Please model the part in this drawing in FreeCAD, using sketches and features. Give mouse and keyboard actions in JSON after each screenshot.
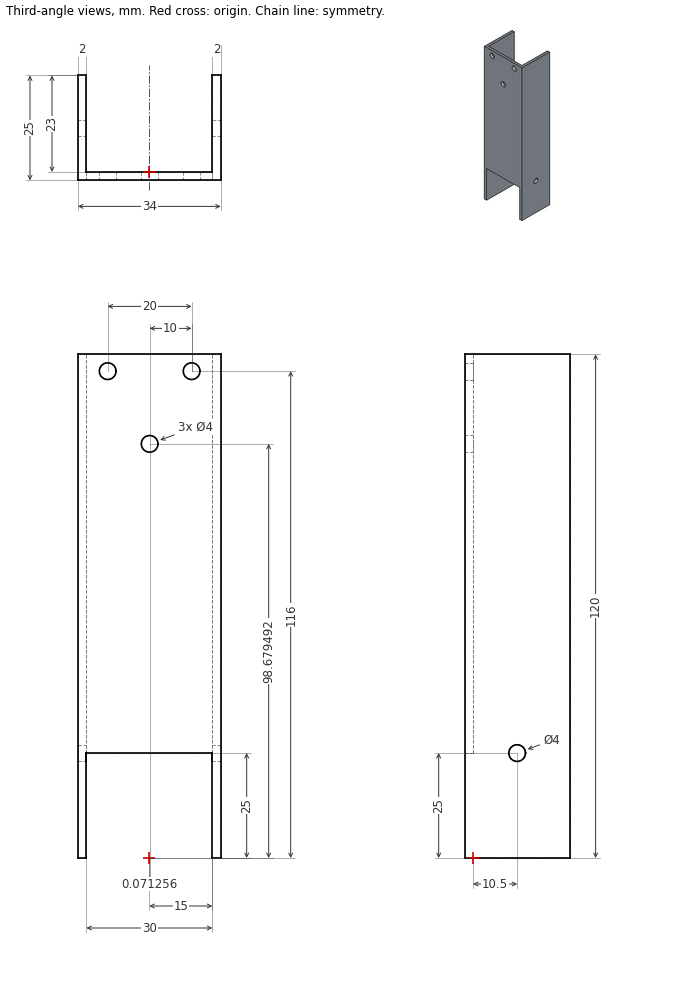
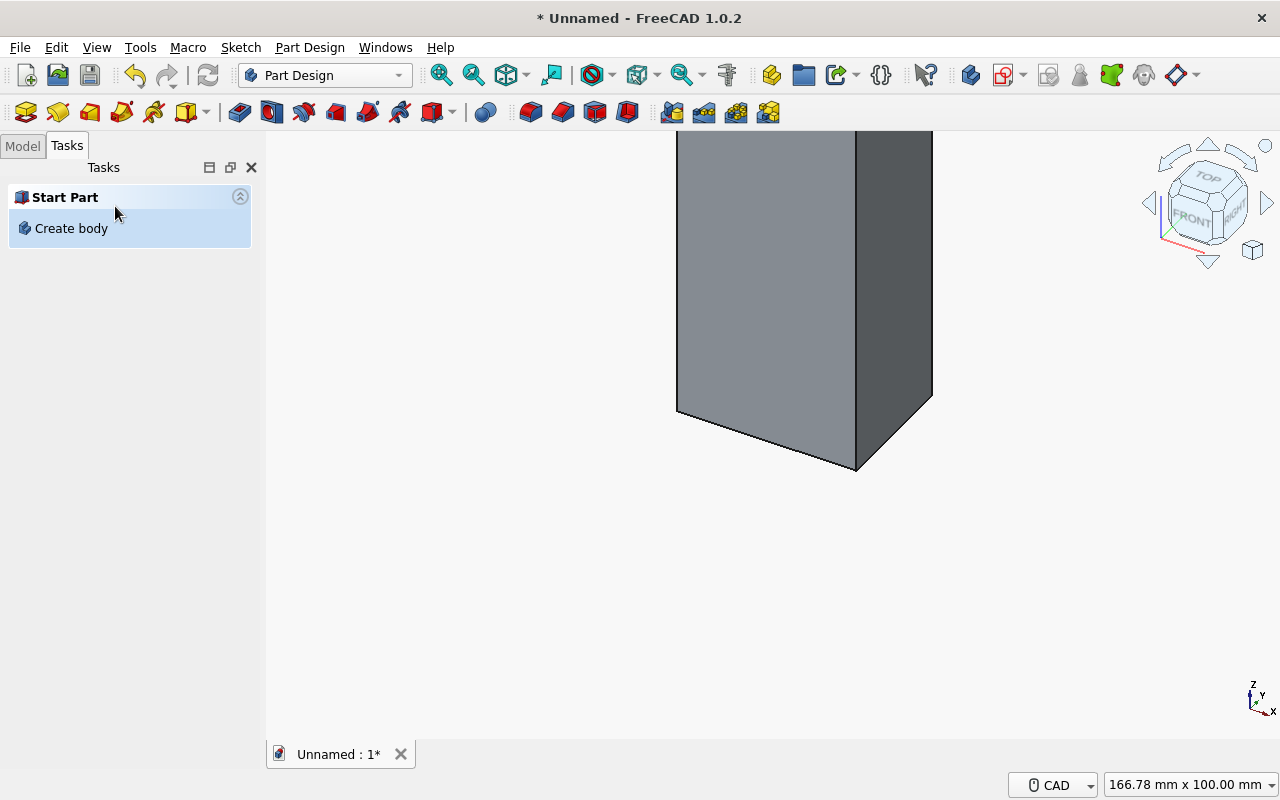
{"action": "left_click", "coordinate": [442, 76]}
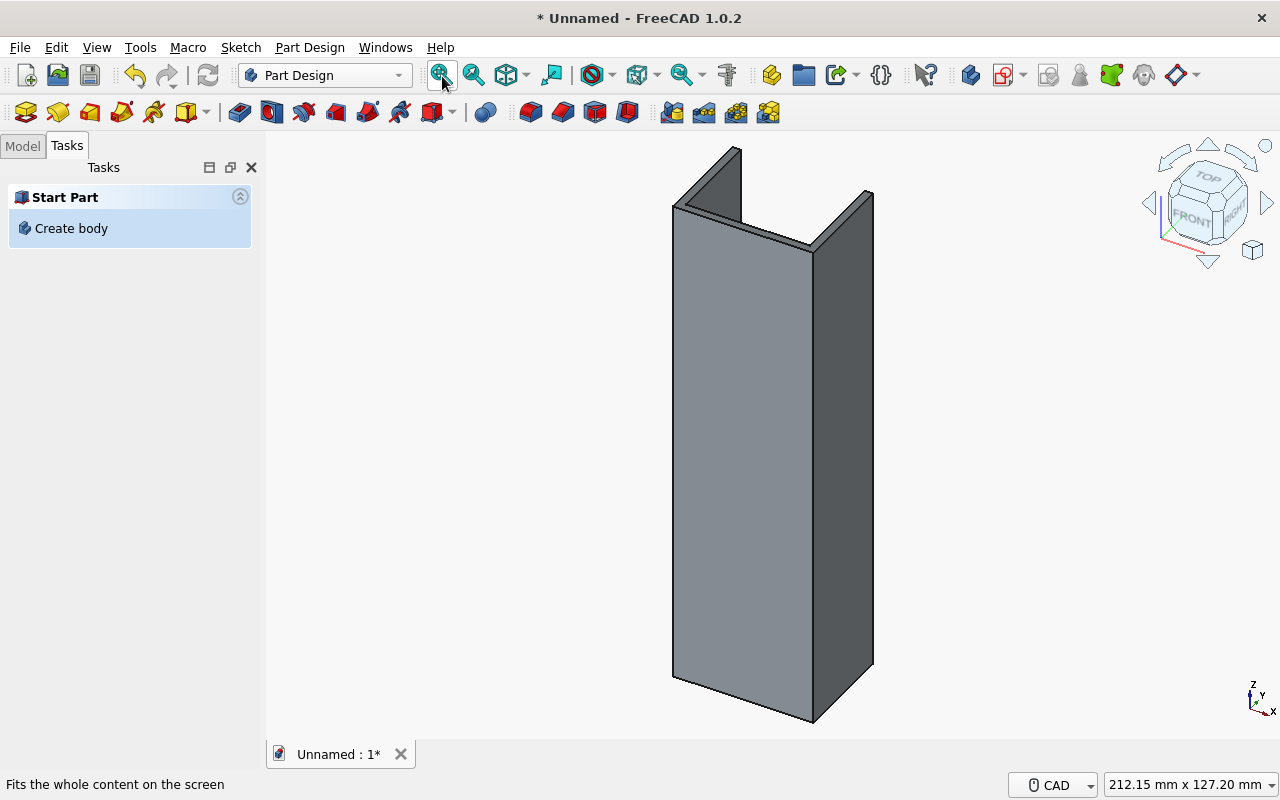
{"action": "left_click", "coordinate": [743, 329]}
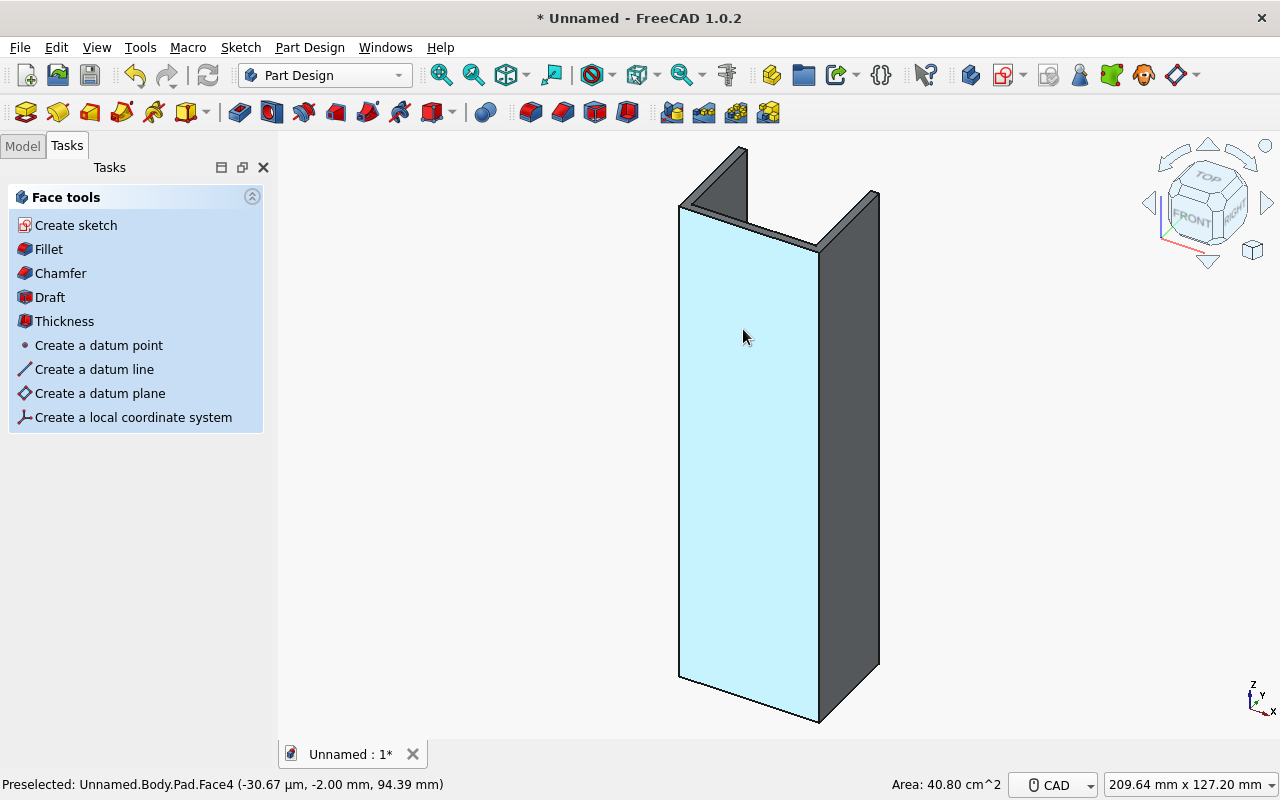
{"action": "left_click", "coordinate": [1004, 76]}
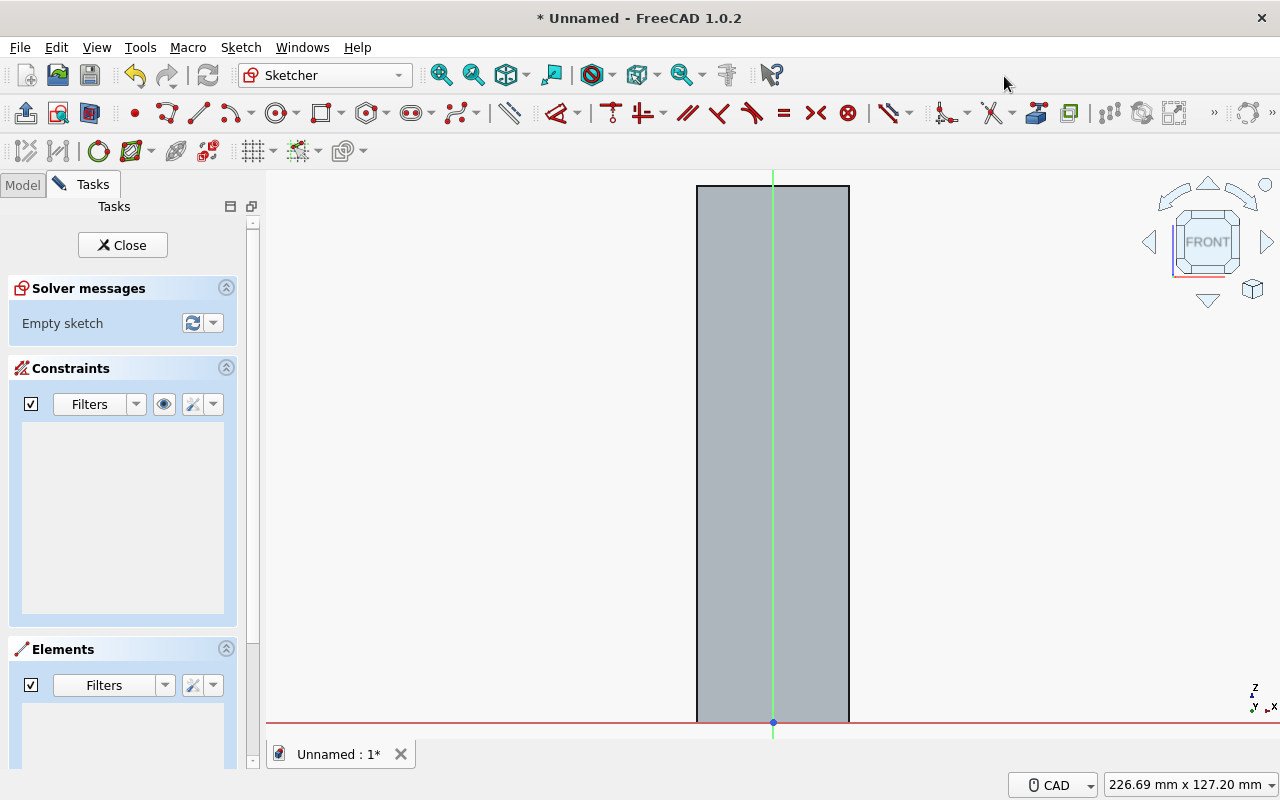
{"action": "scroll", "coordinate": [704, 454], "scroll_direction": "down", "scroll_amount": 5}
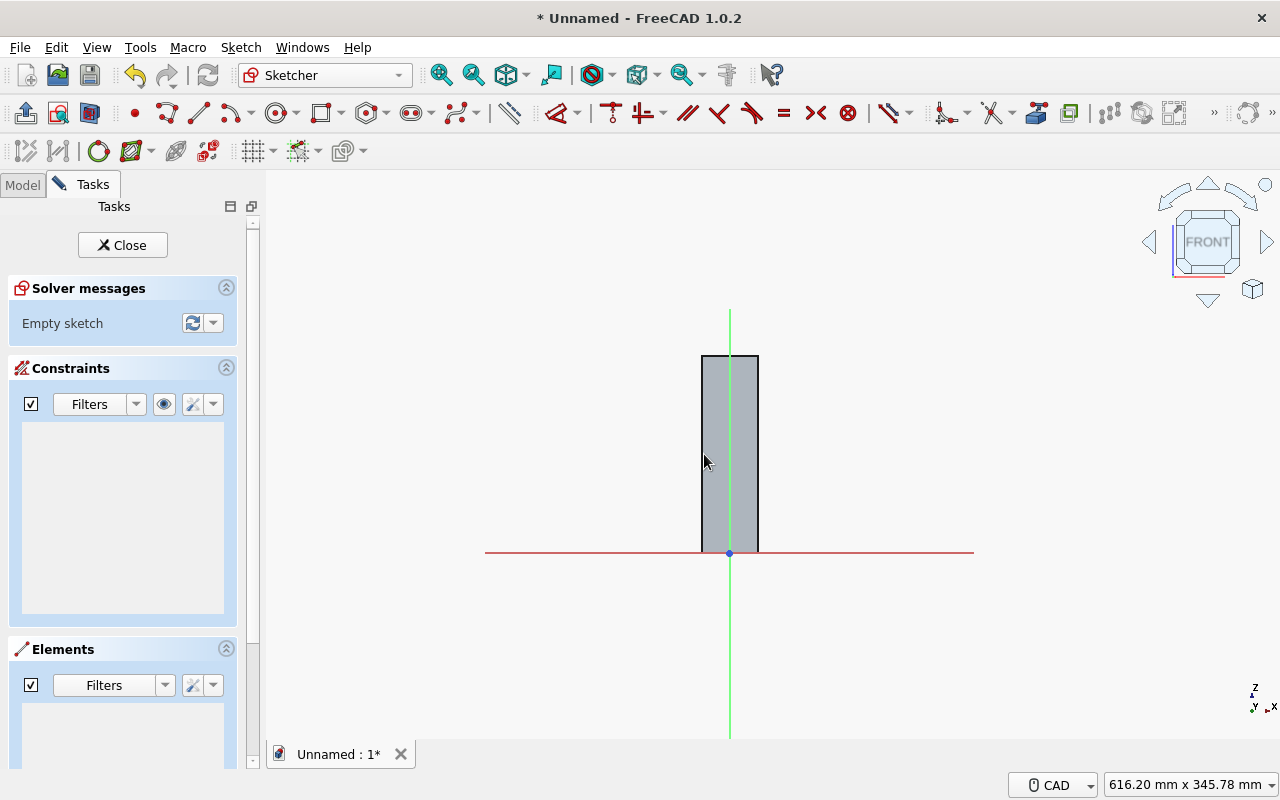
{"action": "scroll", "coordinate": [732, 369], "scroll_direction": "up", "scroll_amount": 12}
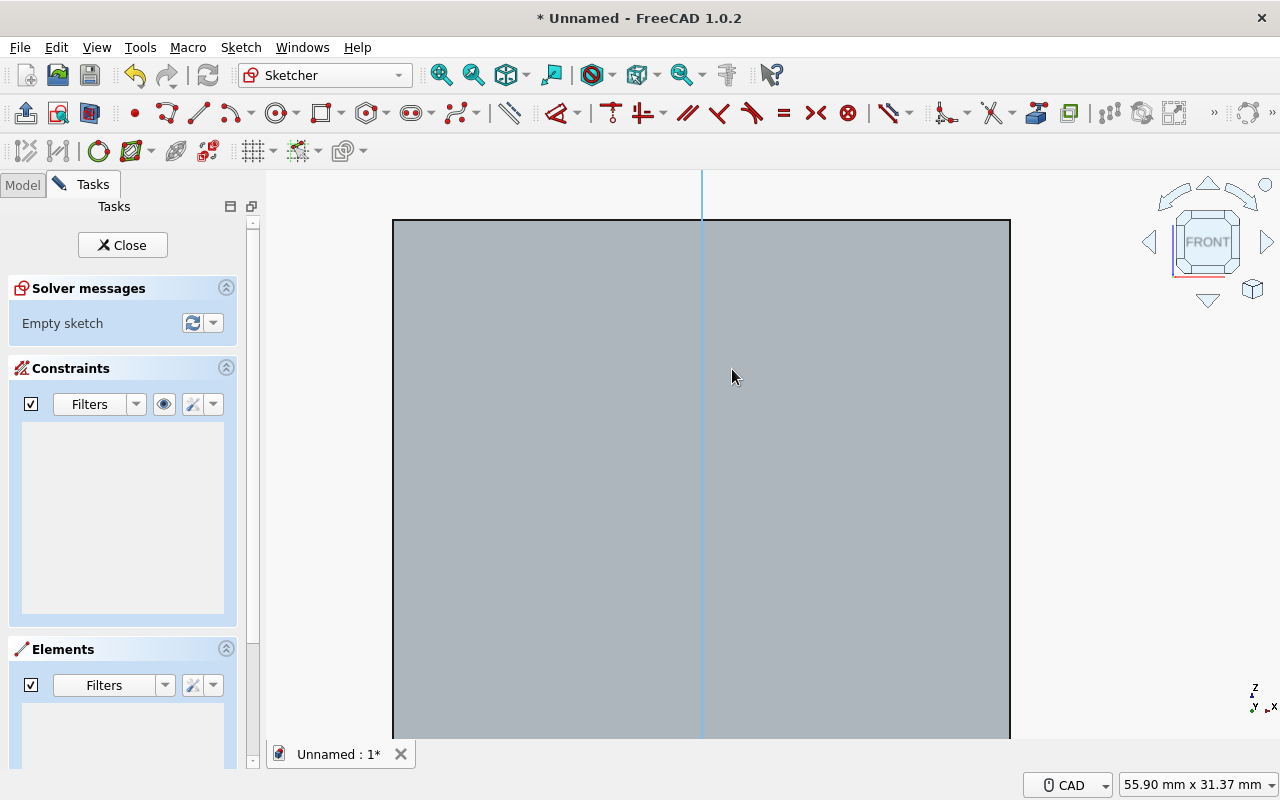
{"action": "left_click", "coordinate": [276, 114]}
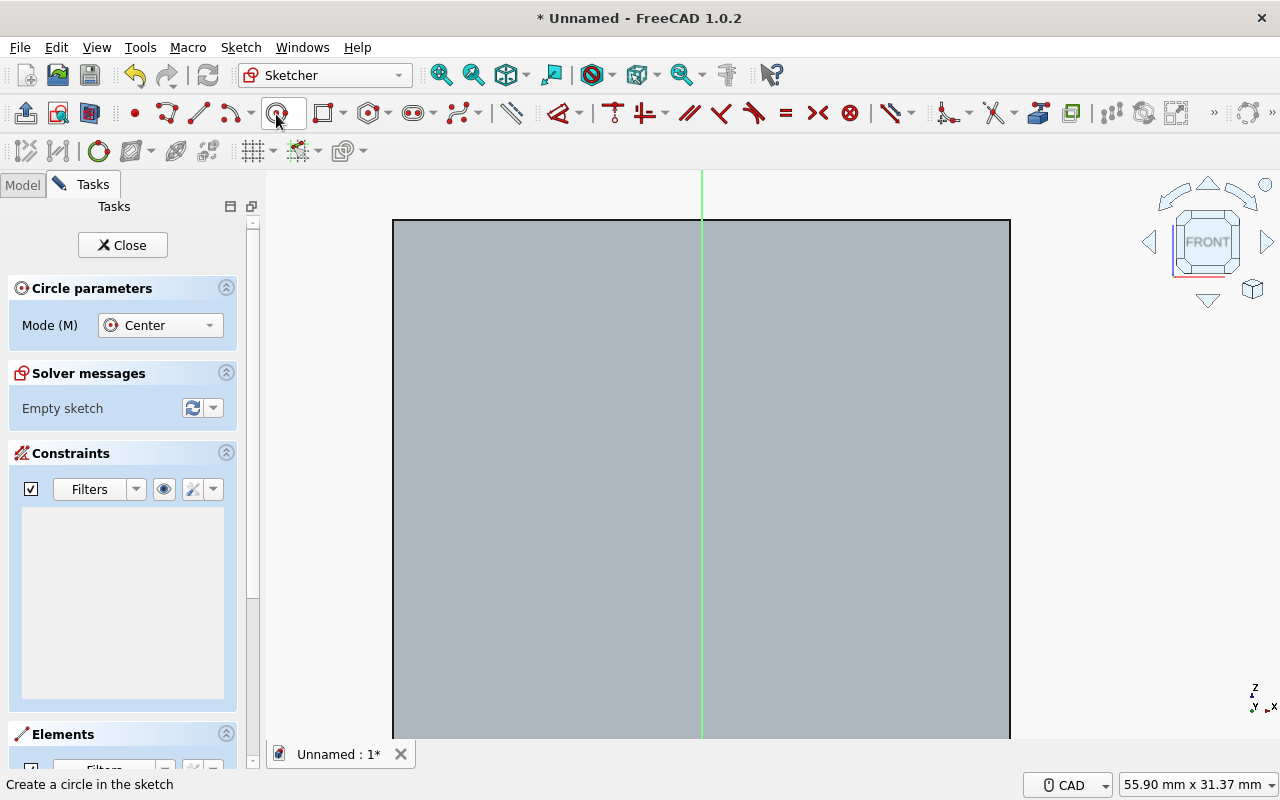
{"action": "scroll", "coordinate": [703, 606], "scroll_direction": "up", "scroll_amount": 13}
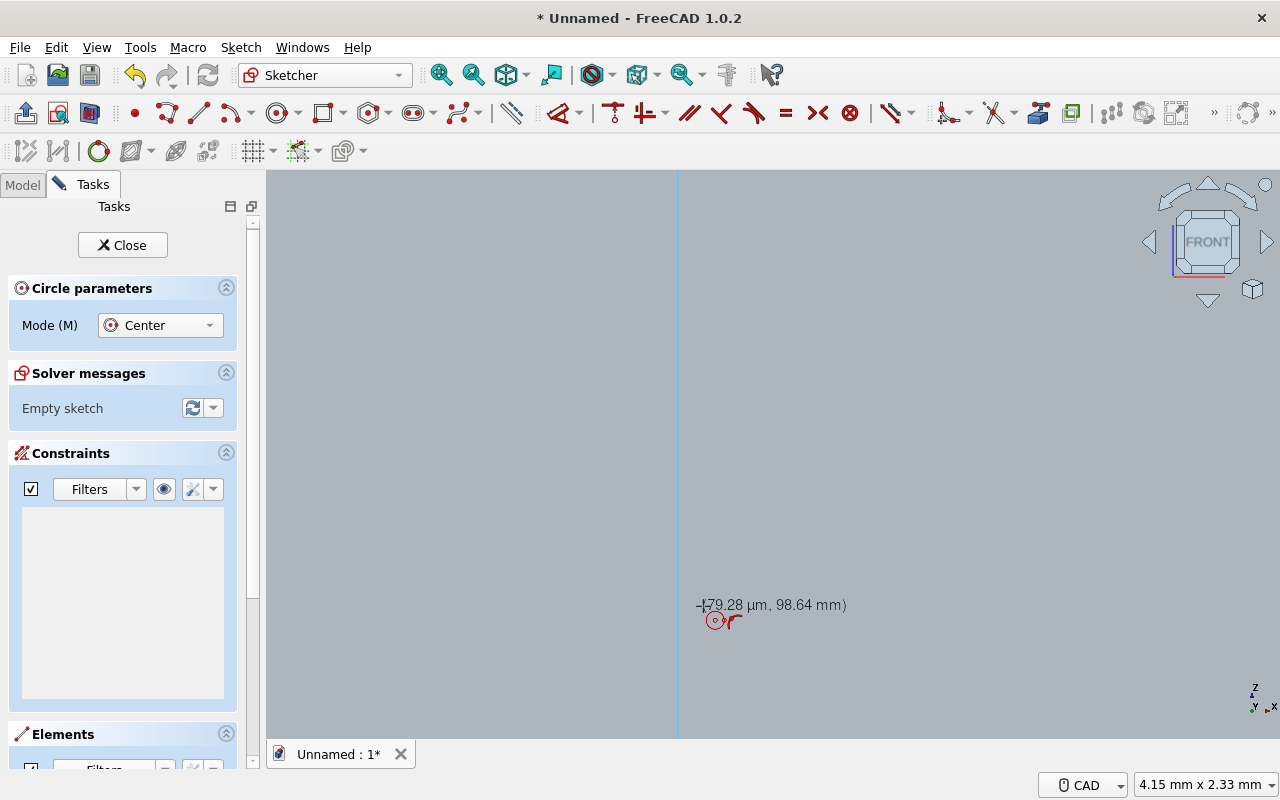
{"action": "left_click", "coordinate": [696, 601]}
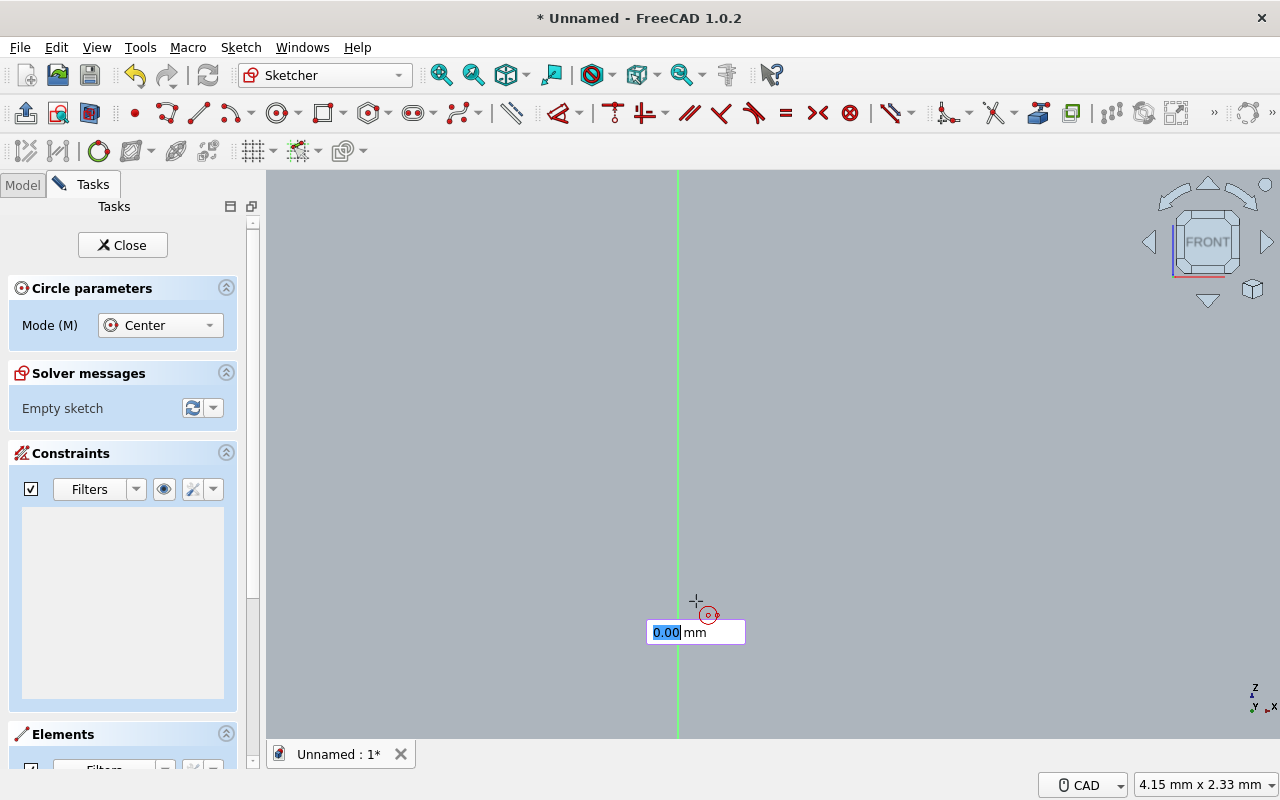
{"action": "scroll", "coordinate": [705, 612], "scroll_direction": "down", "scroll_amount": 13}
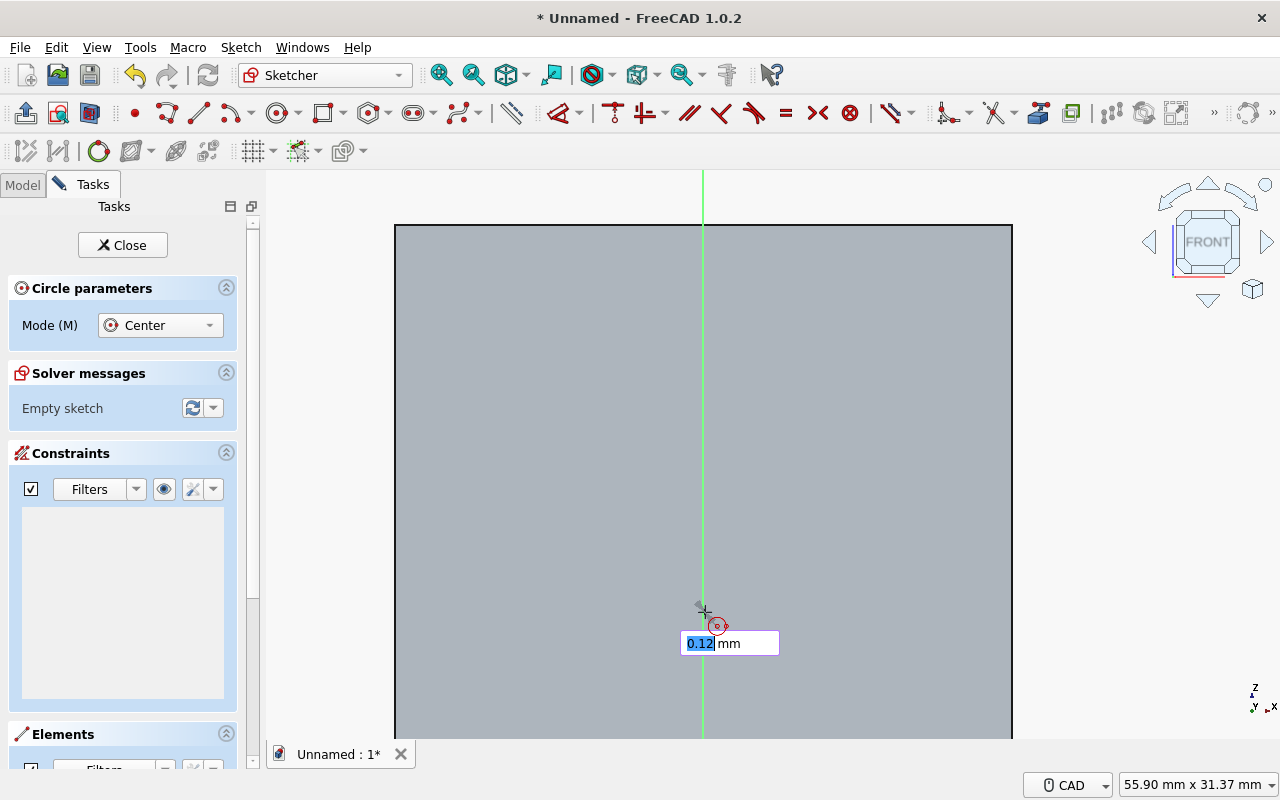
{"action": "left_click", "coordinate": [730, 586]}